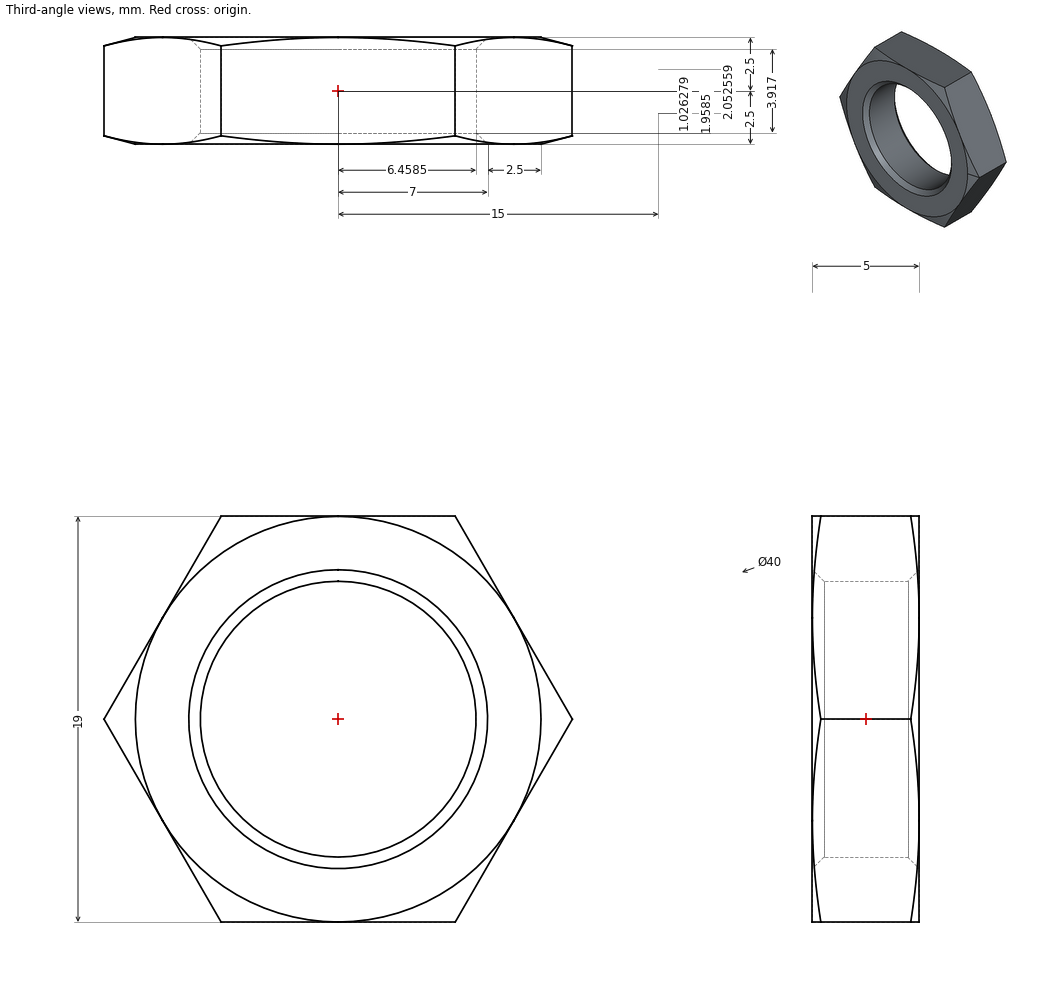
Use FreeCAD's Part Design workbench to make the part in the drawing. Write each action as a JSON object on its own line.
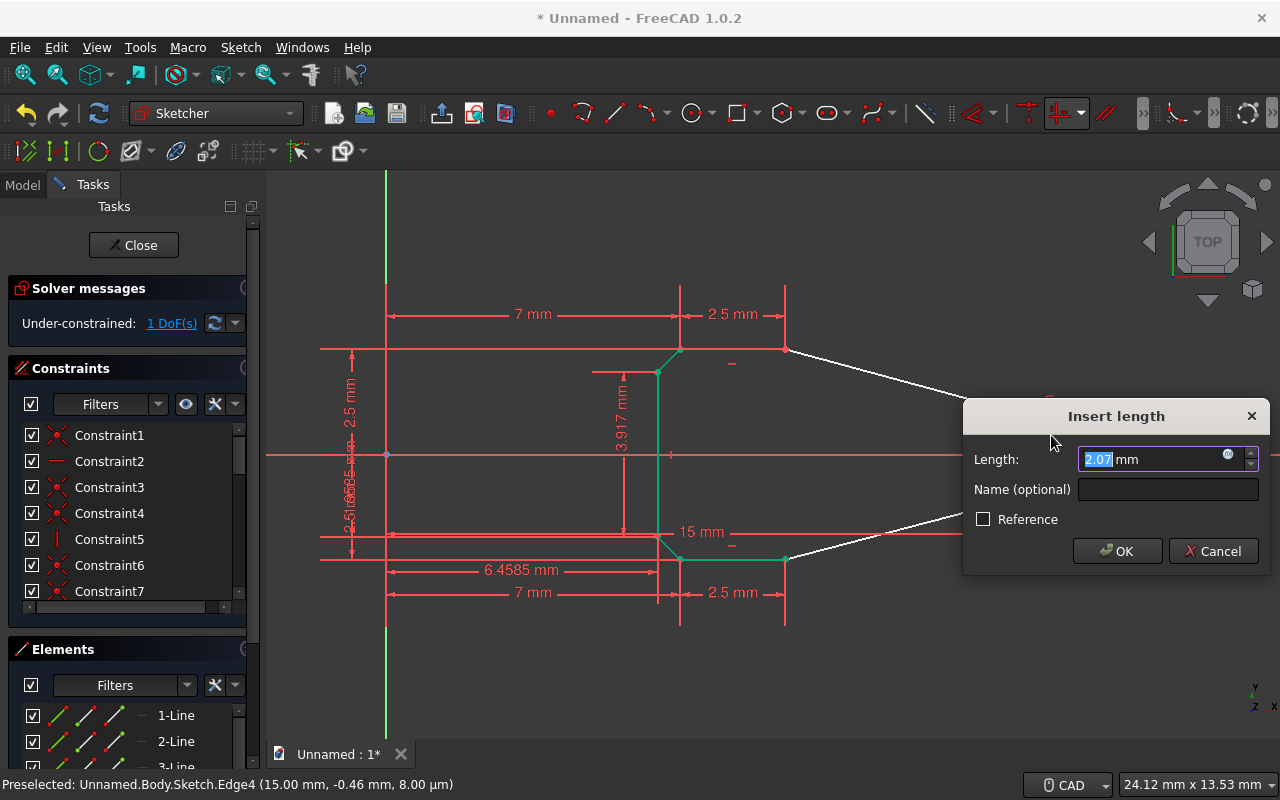
{"action": "type", "text": "2.052559"}
{"action": "key", "text": "Return"}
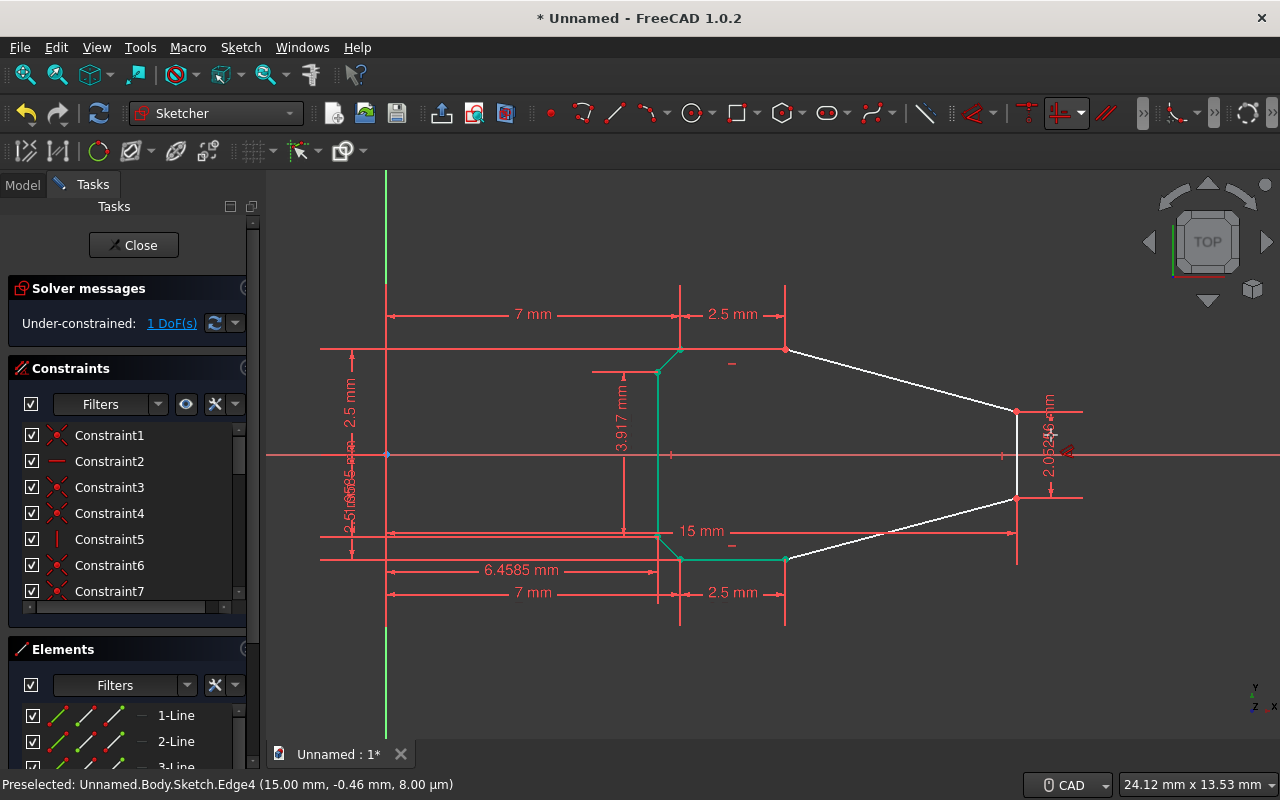
{"action": "left_click", "coordinate": [1017, 498]}
{"action": "left_click", "coordinate": [1051, 476]}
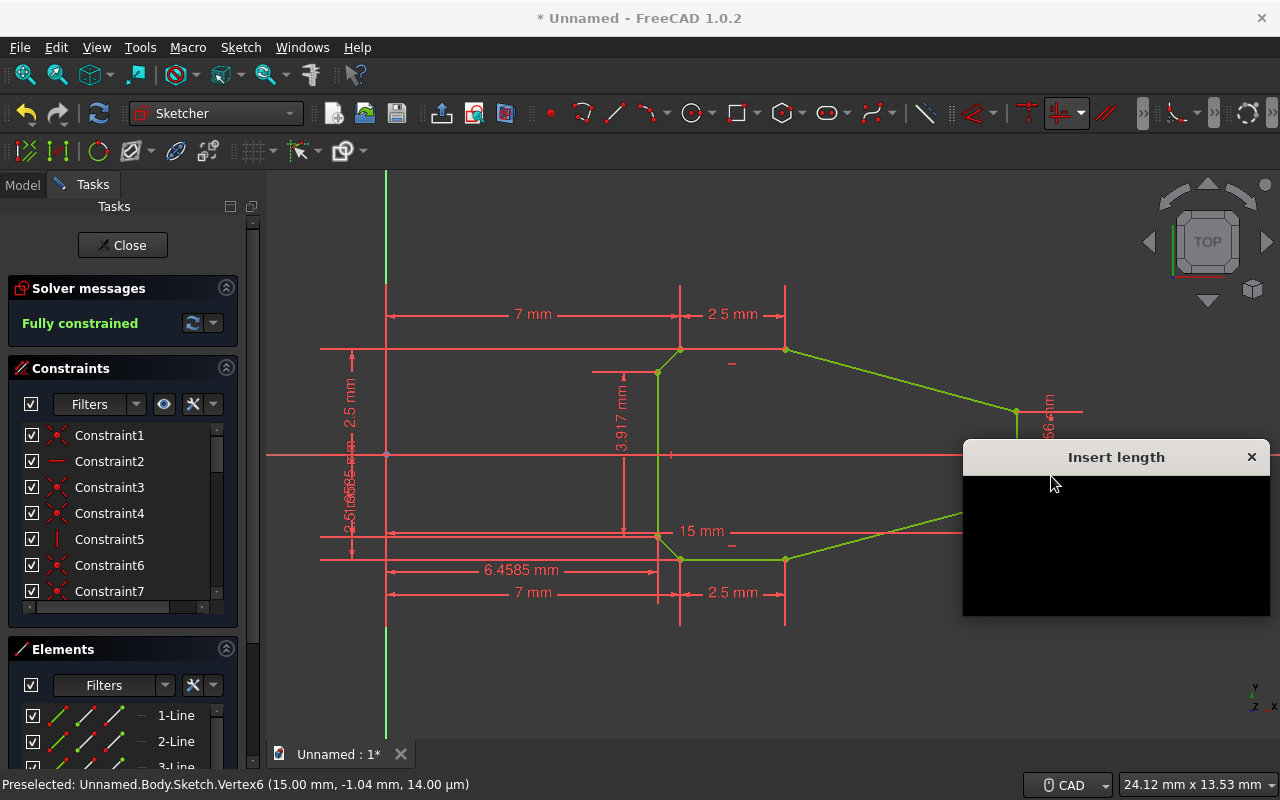
{"action": "type", "text": "1.026279"}
{"action": "key", "text": "Return"}
{"action": "key", "text": "Escape"}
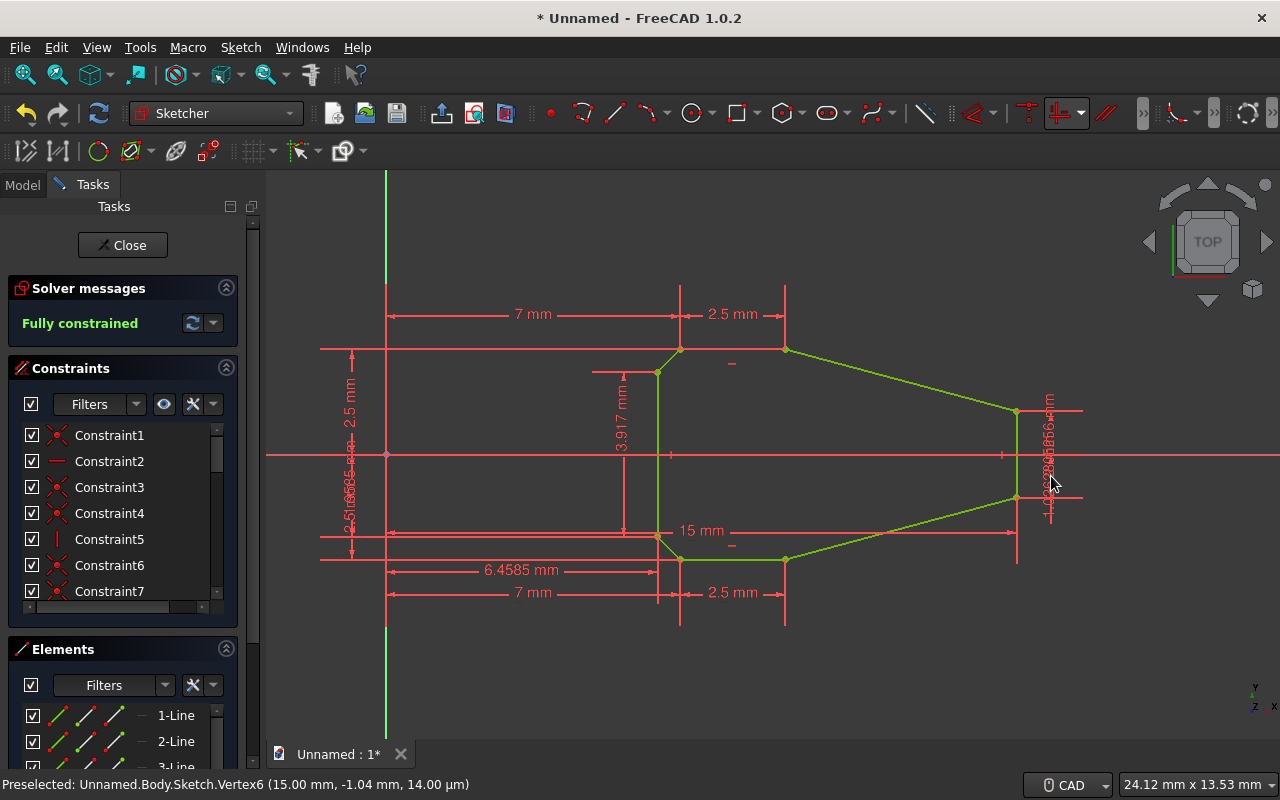
{"action": "left_click", "coordinate": [123, 245]}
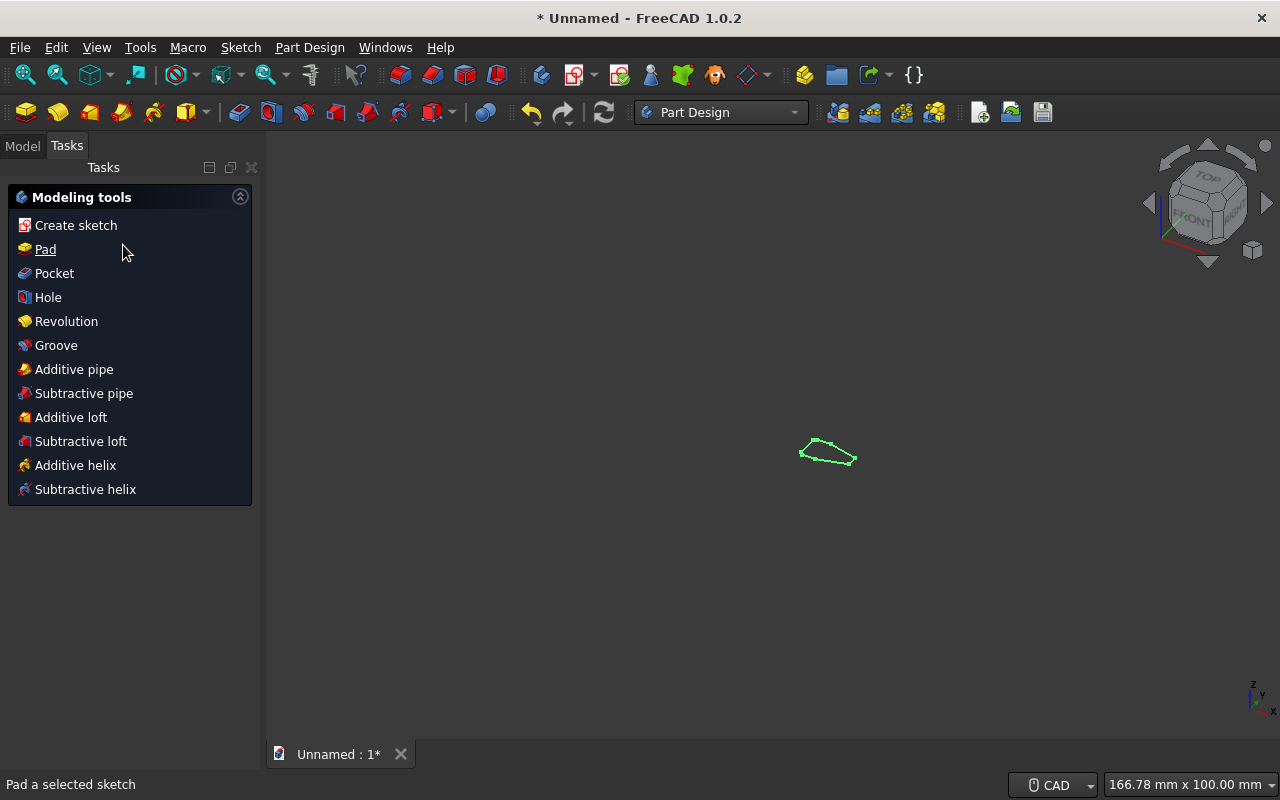
{"action": "left_click", "coordinate": [58, 112]}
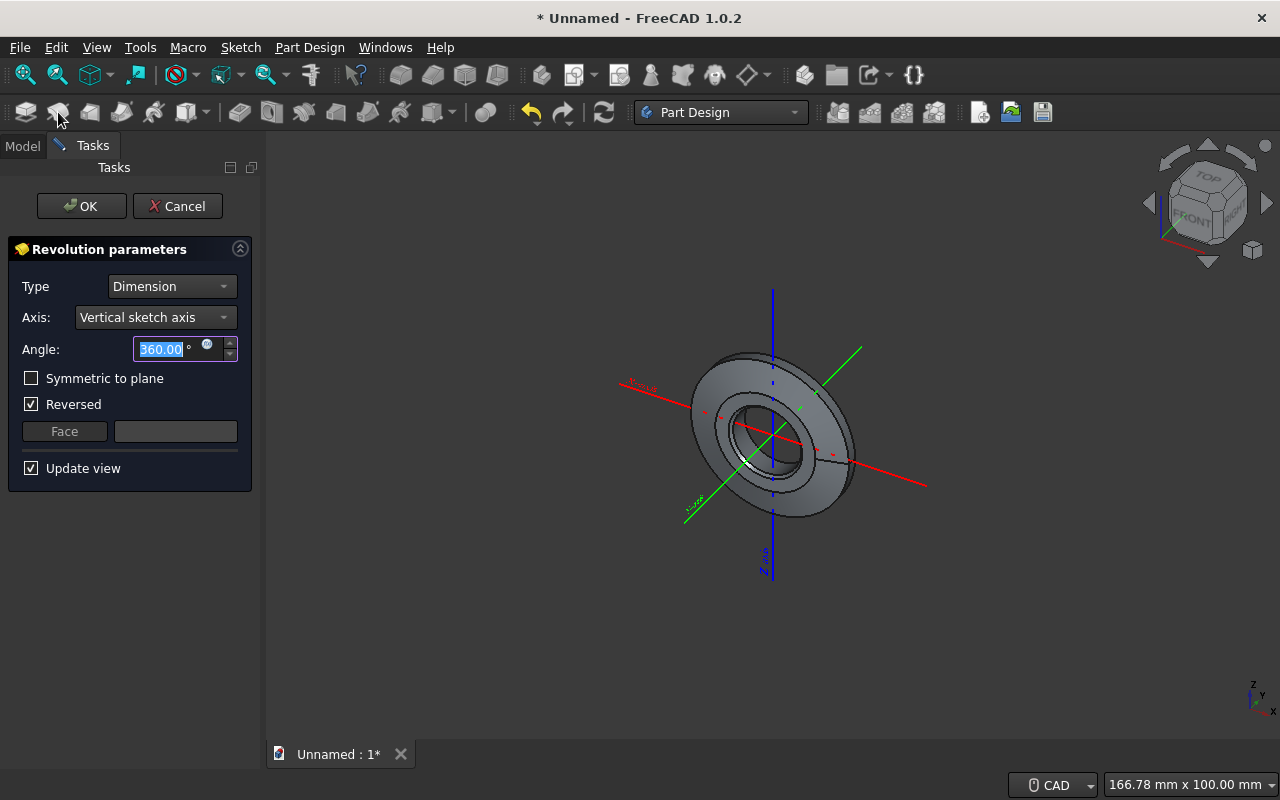
{"action": "left_click", "coordinate": [82, 206]}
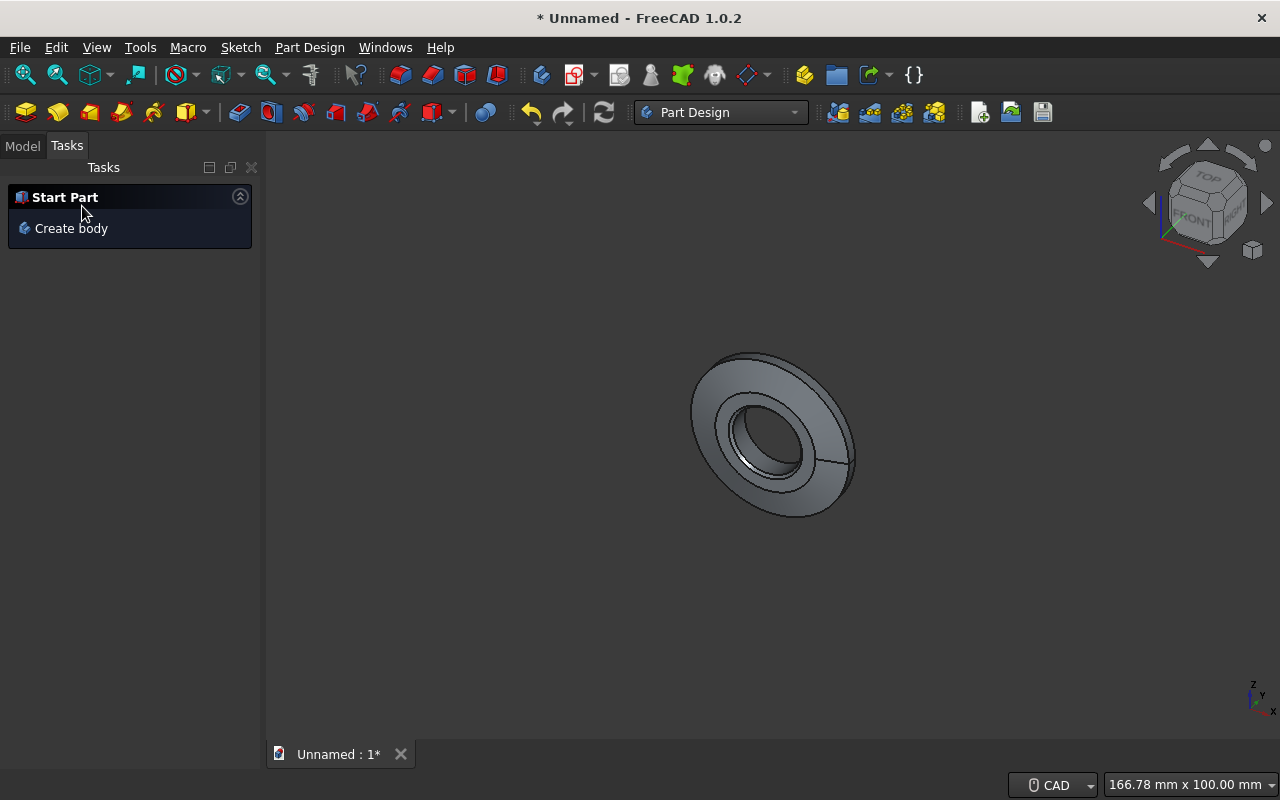
{"action": "left_click", "coordinate": [26, 76]}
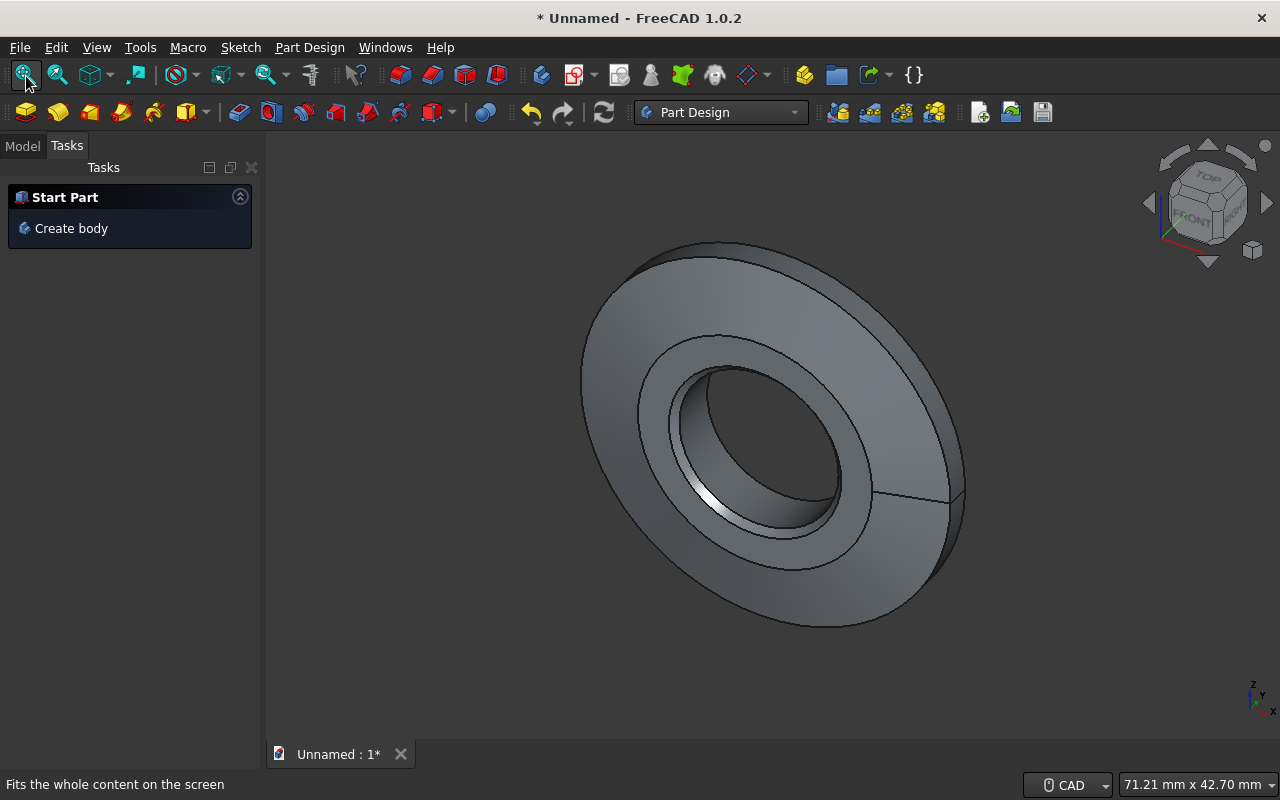
{"action": "left_click", "coordinate": [574, 76]}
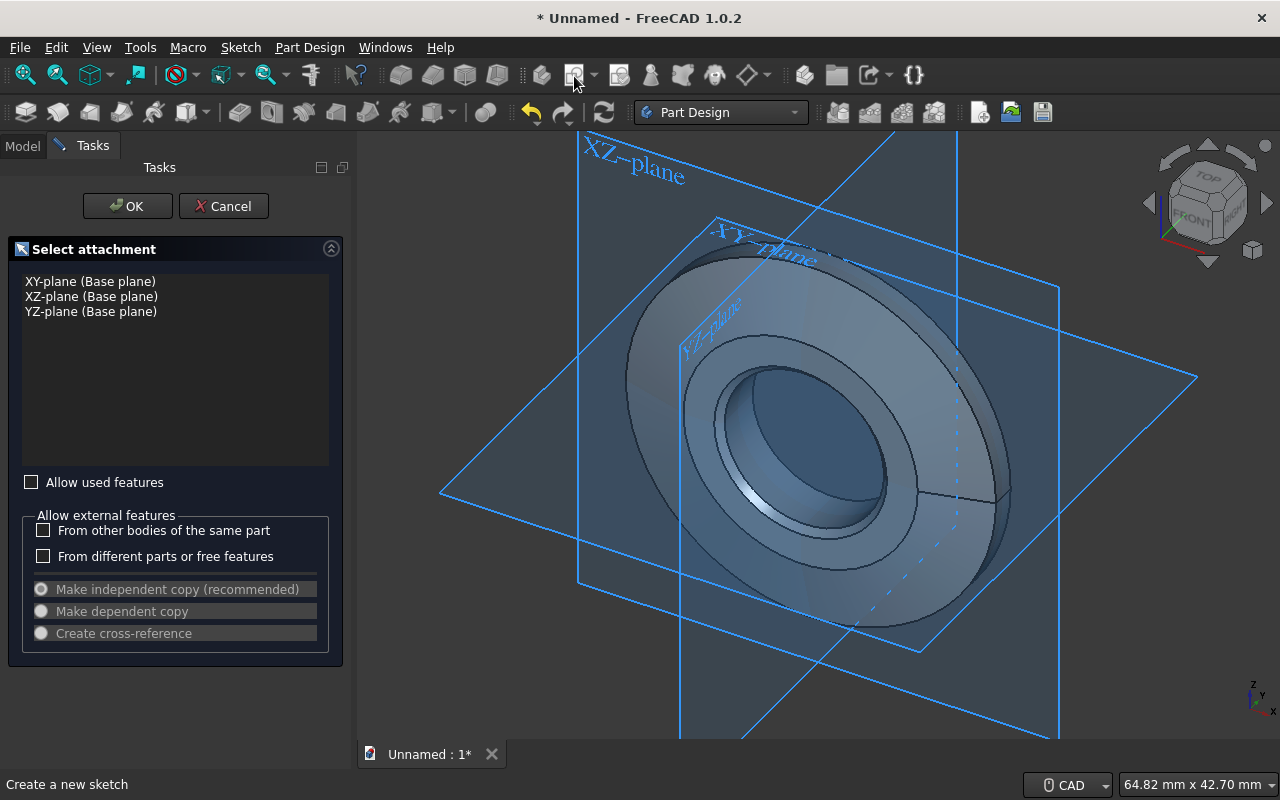
{"action": "left_click", "coordinate": [82, 296]}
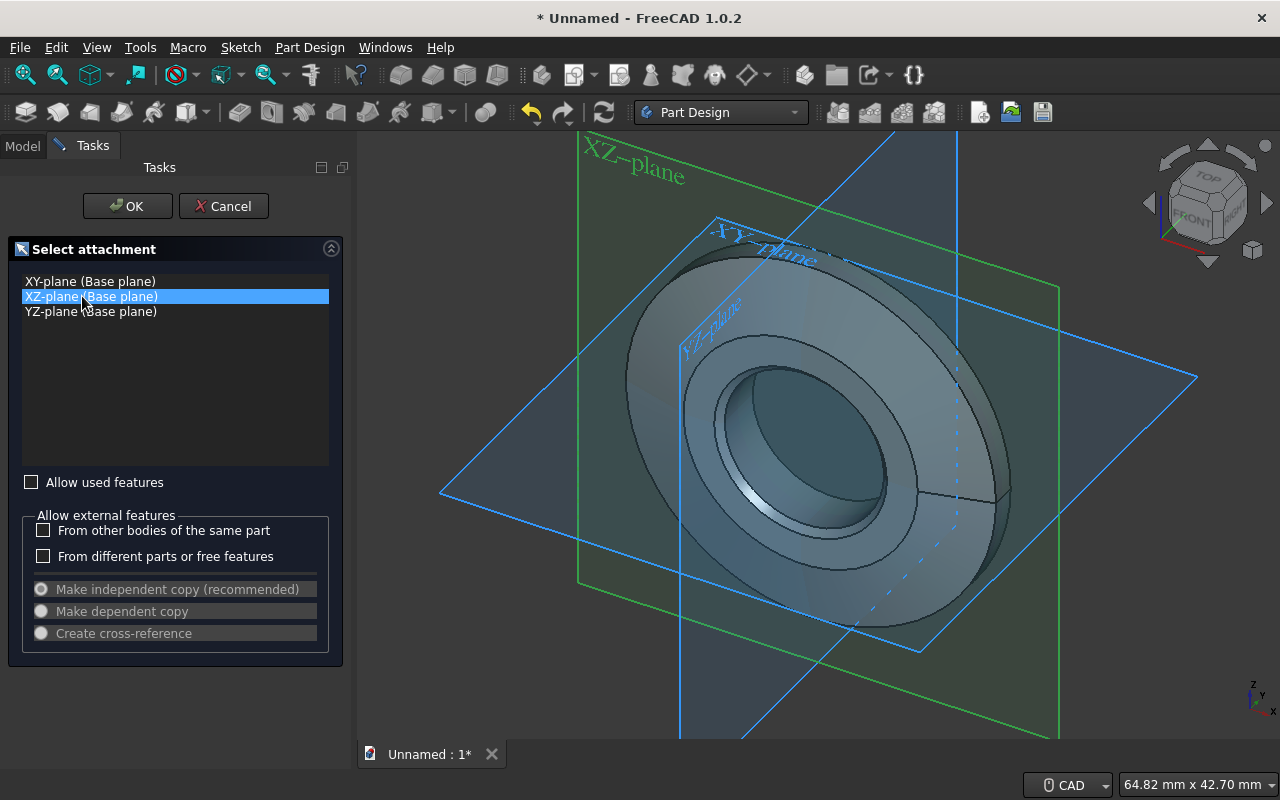
{"action": "left_click", "coordinate": [128, 206]}